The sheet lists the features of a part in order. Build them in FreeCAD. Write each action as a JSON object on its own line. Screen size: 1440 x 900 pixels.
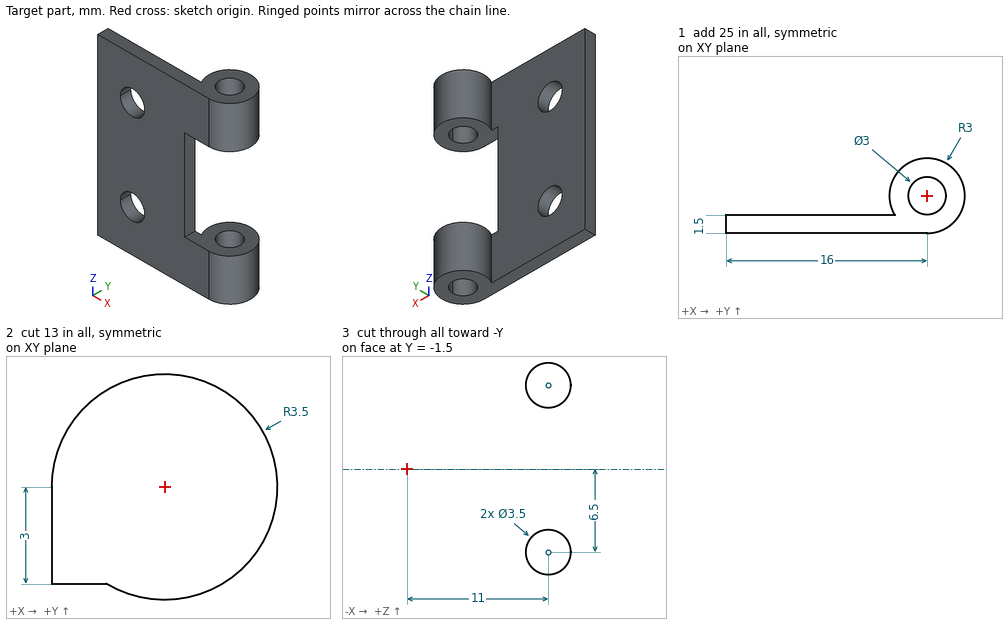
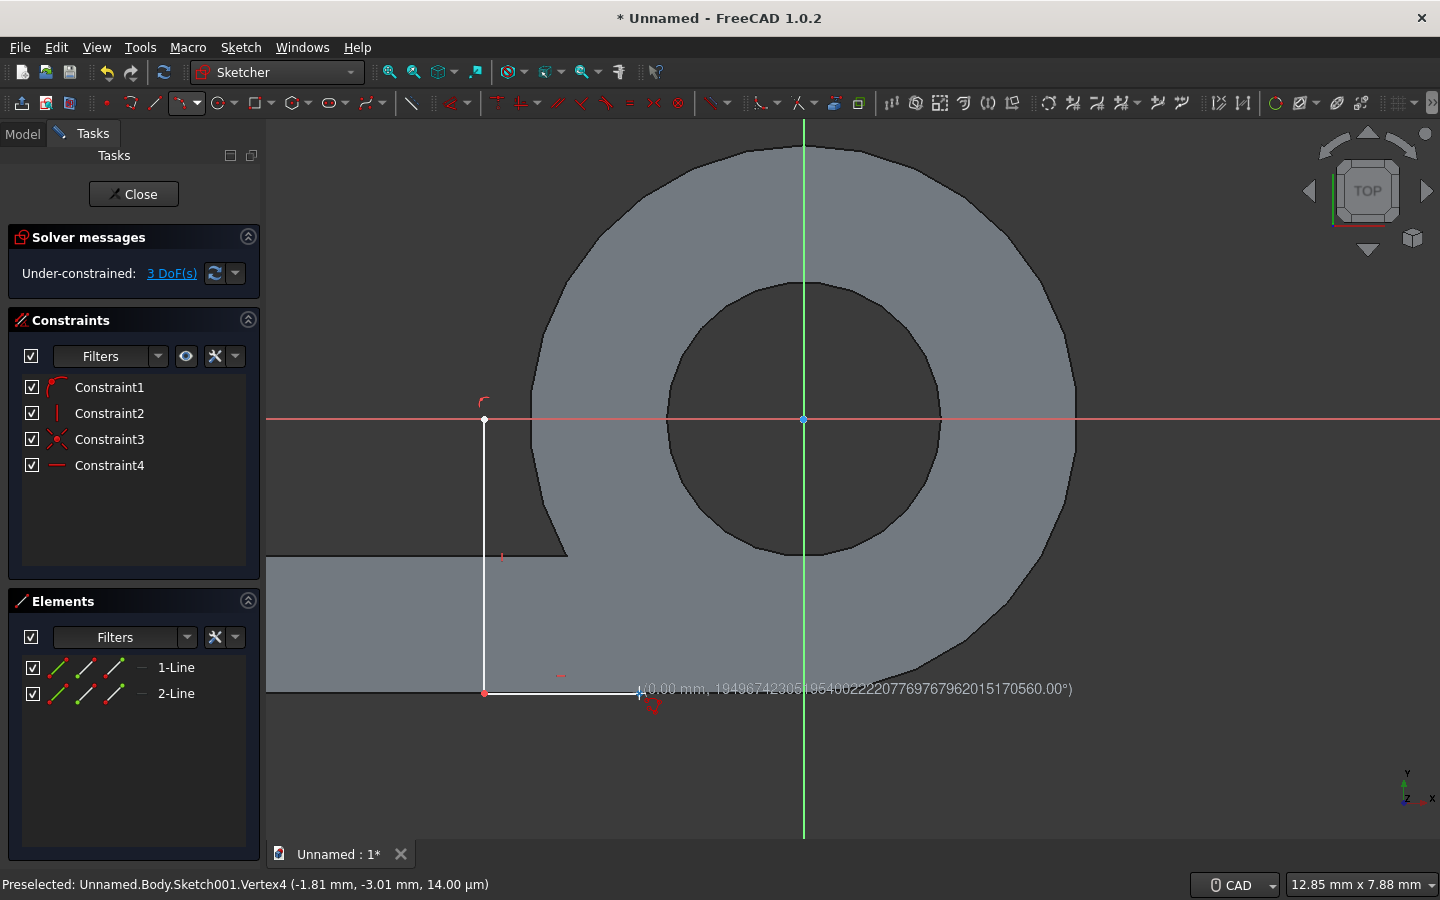
{"action": "left_click", "coordinate": [180, 104]}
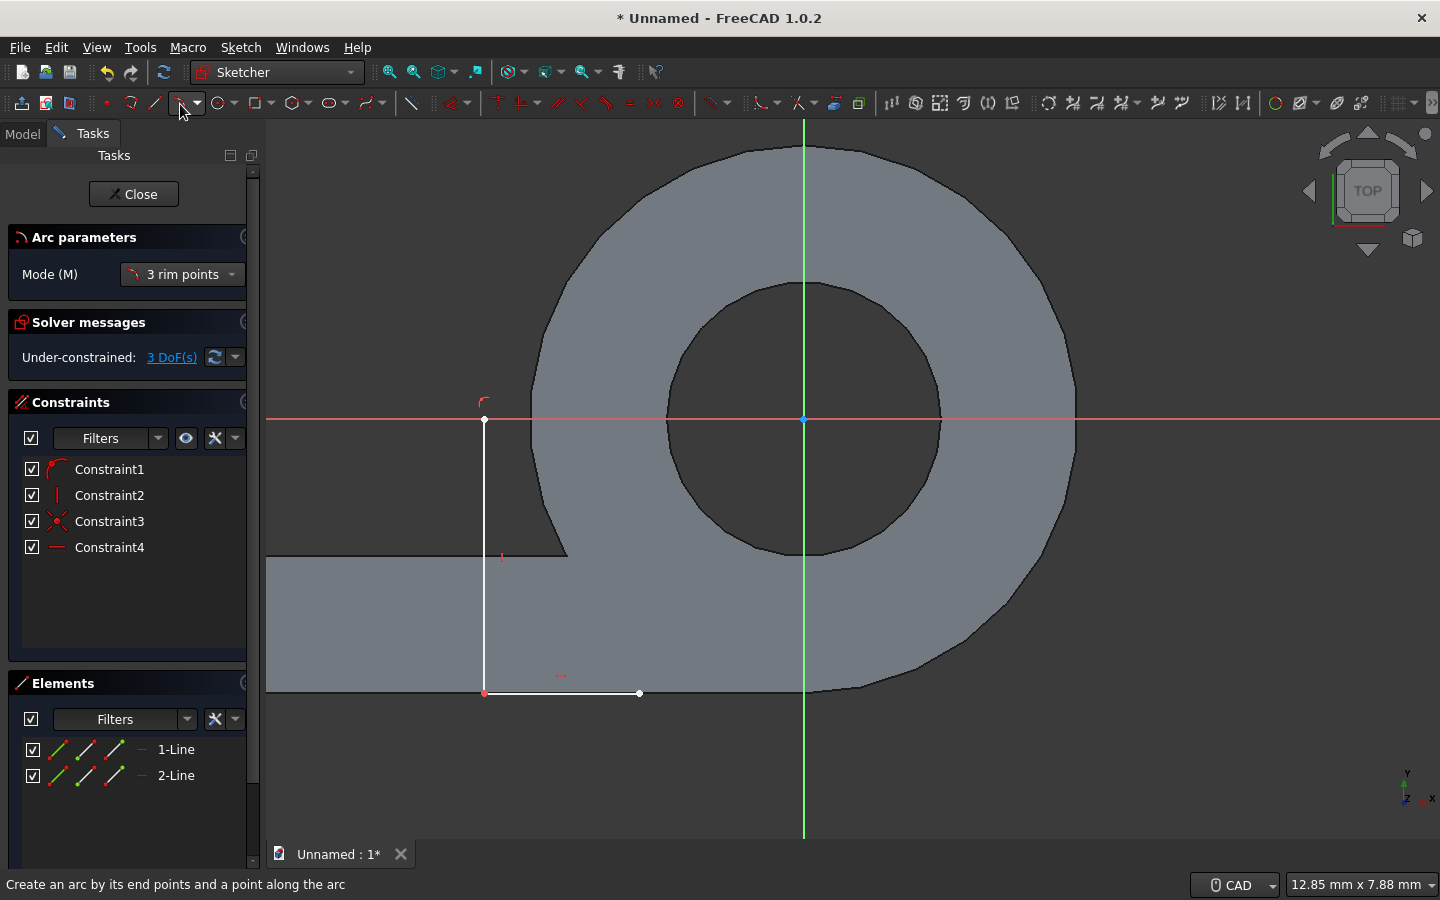
{"action": "left_click", "coordinate": [639, 694]}
{"action": "left_click", "coordinate": [484, 419]}
{"action": "left_click", "coordinate": [1082, 262]}
{"action": "key", "text": "Escape"}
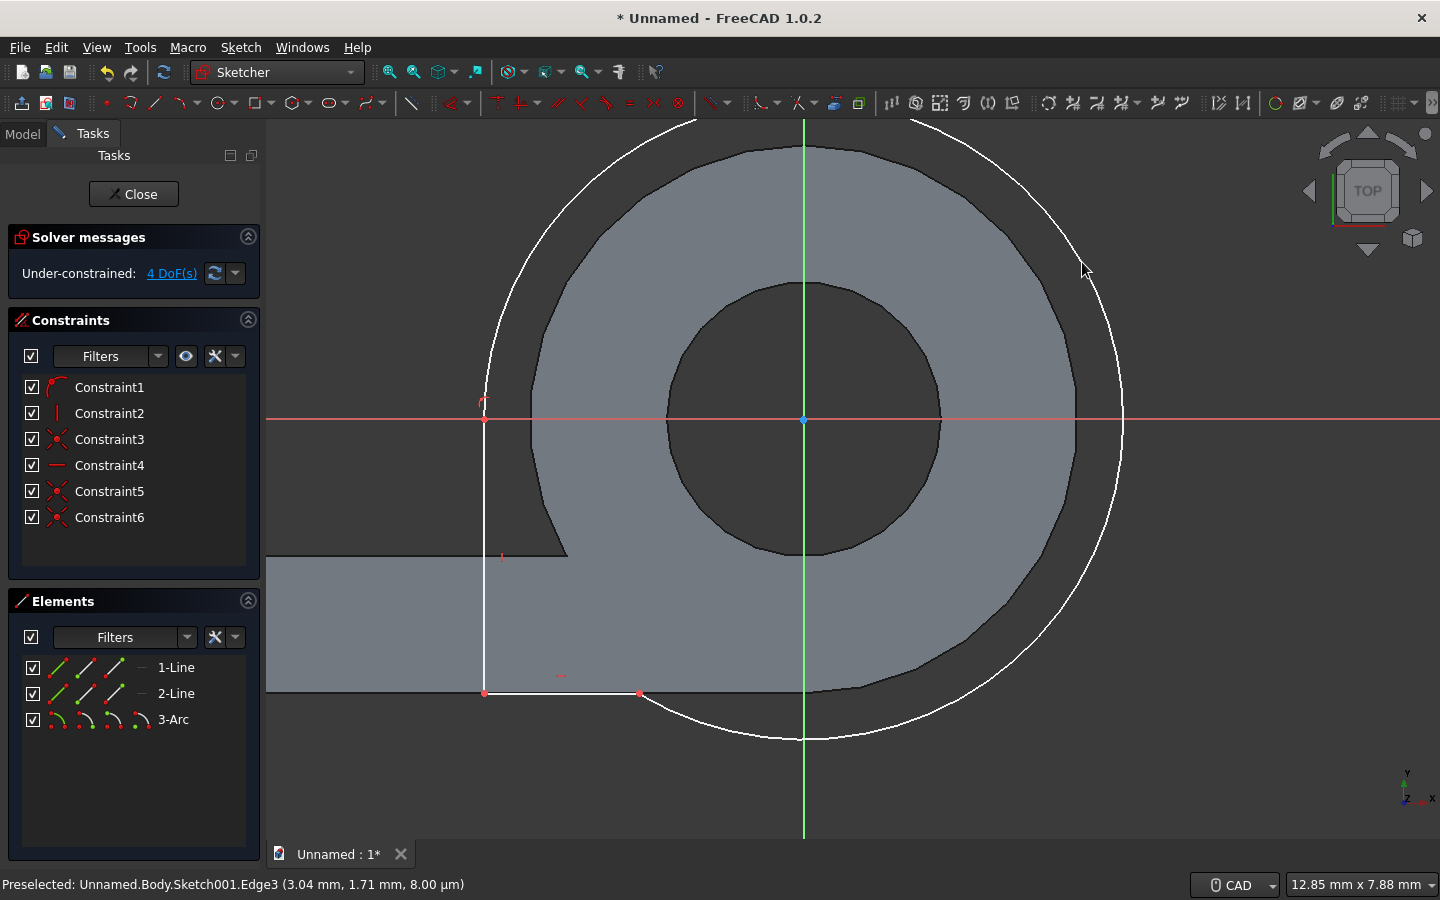
{"action": "left_click", "coordinate": [484, 502]}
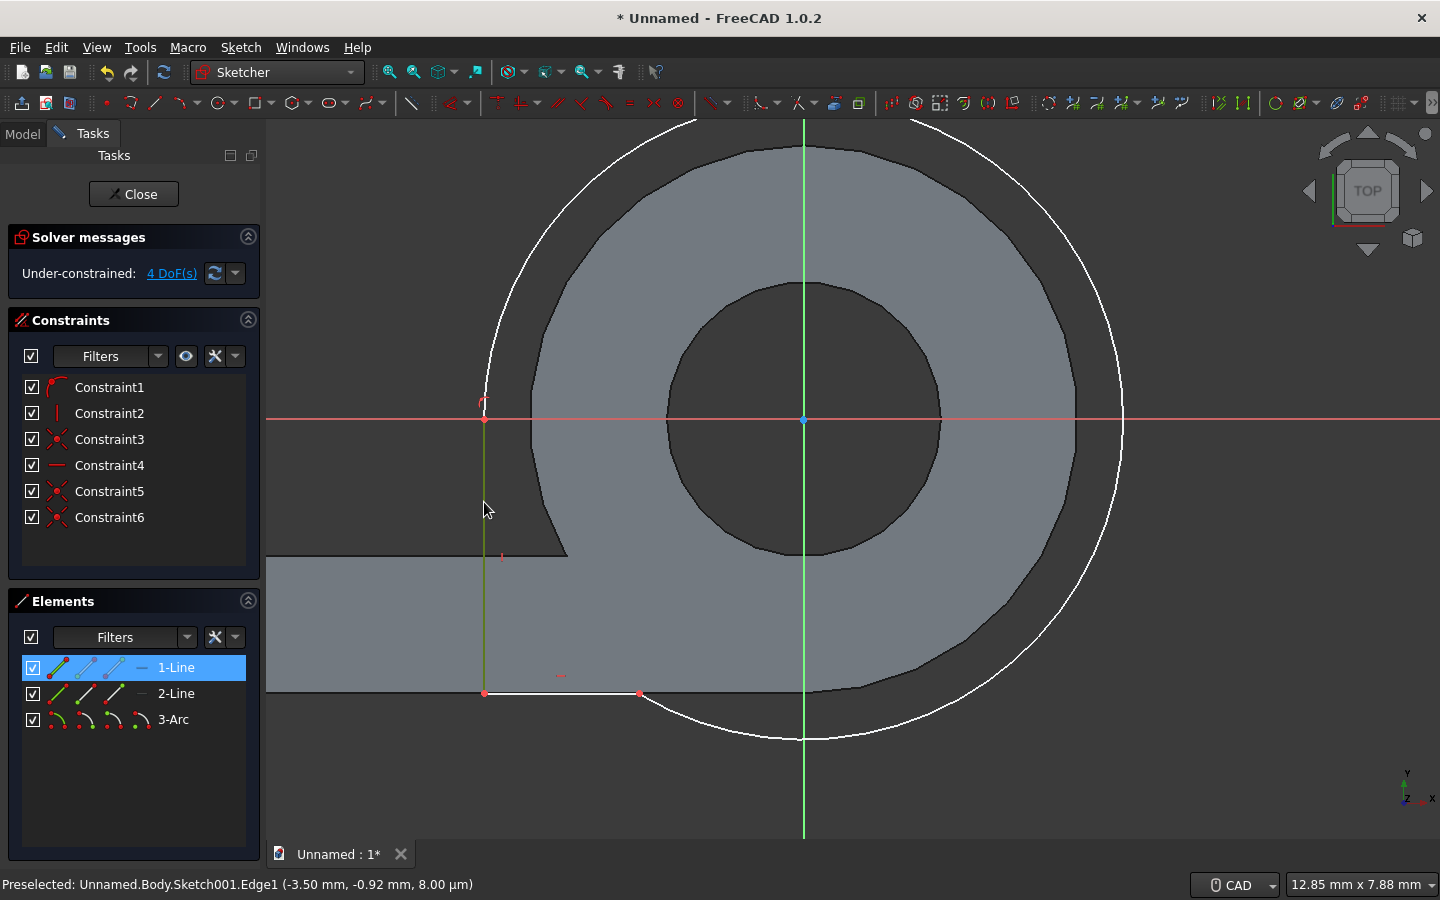
{"action": "left_click", "coordinate": [1078, 583]}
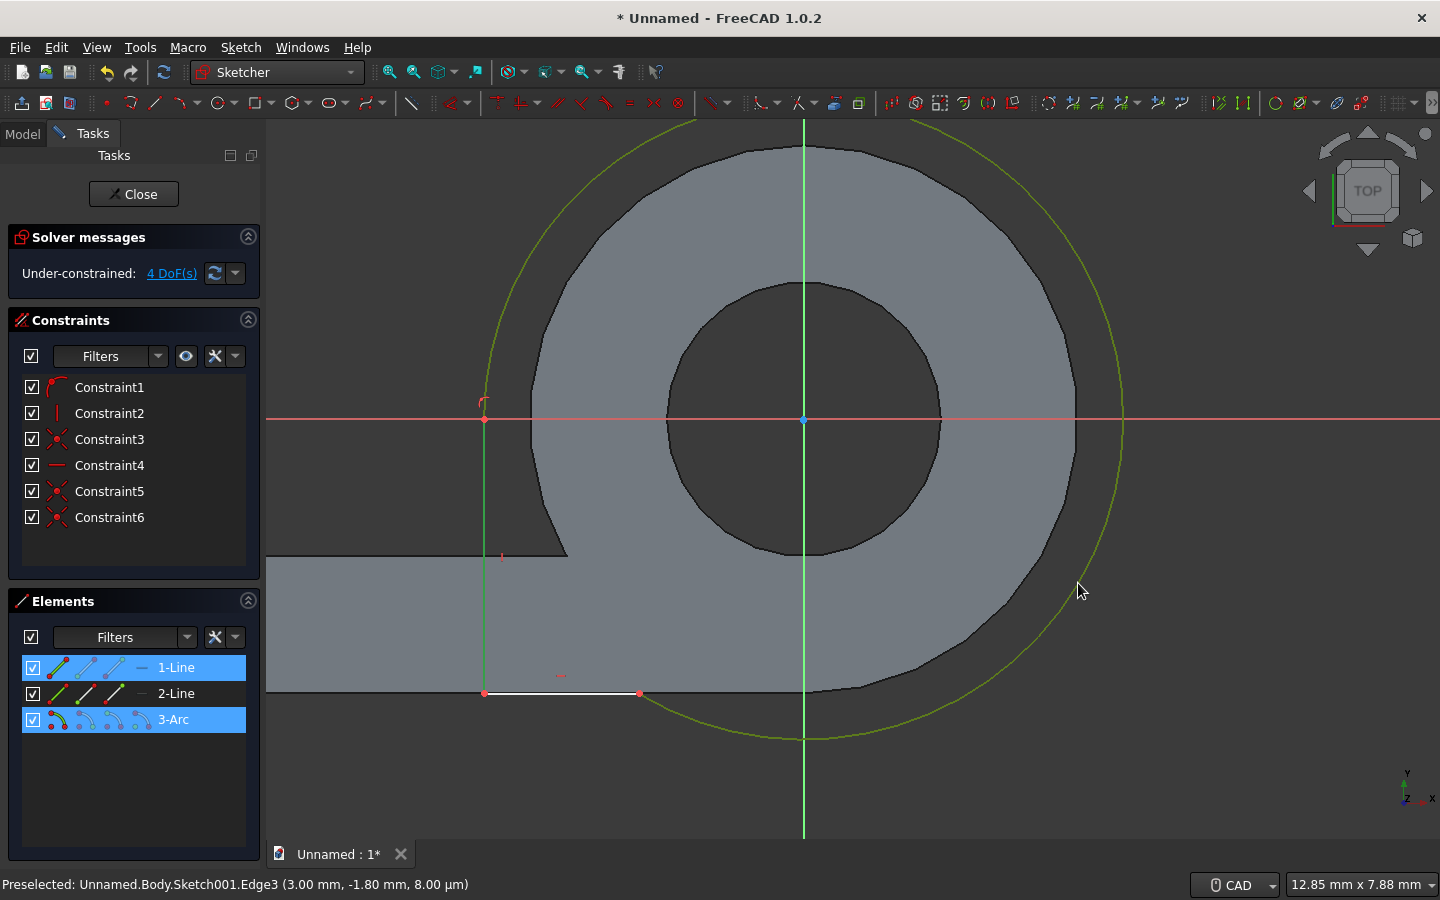
{"action": "left_click", "coordinate": [606, 104]}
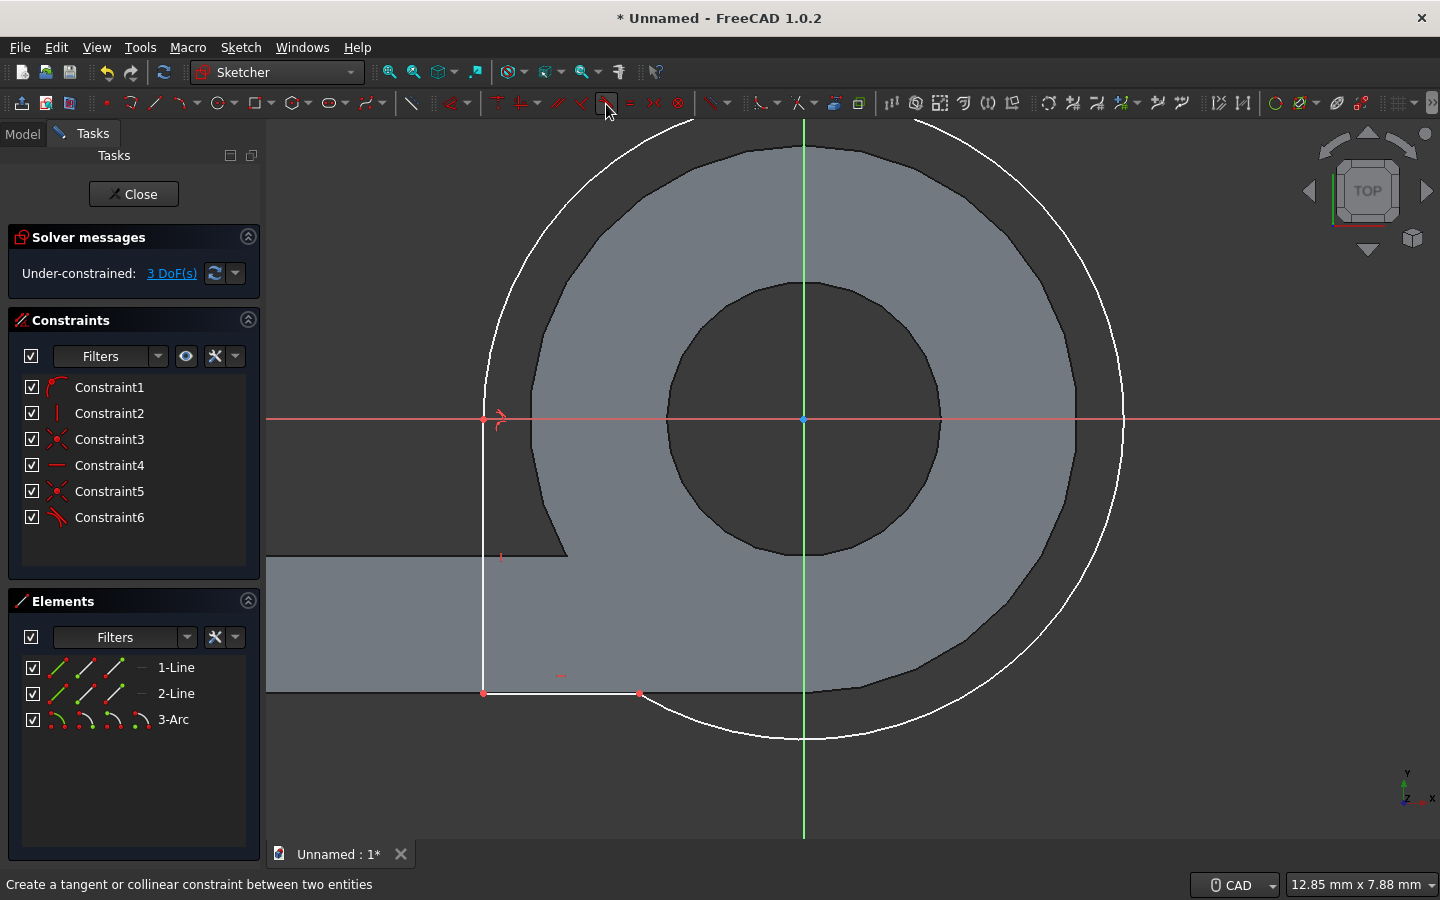
{"action": "left_click", "coordinate": [804, 419]}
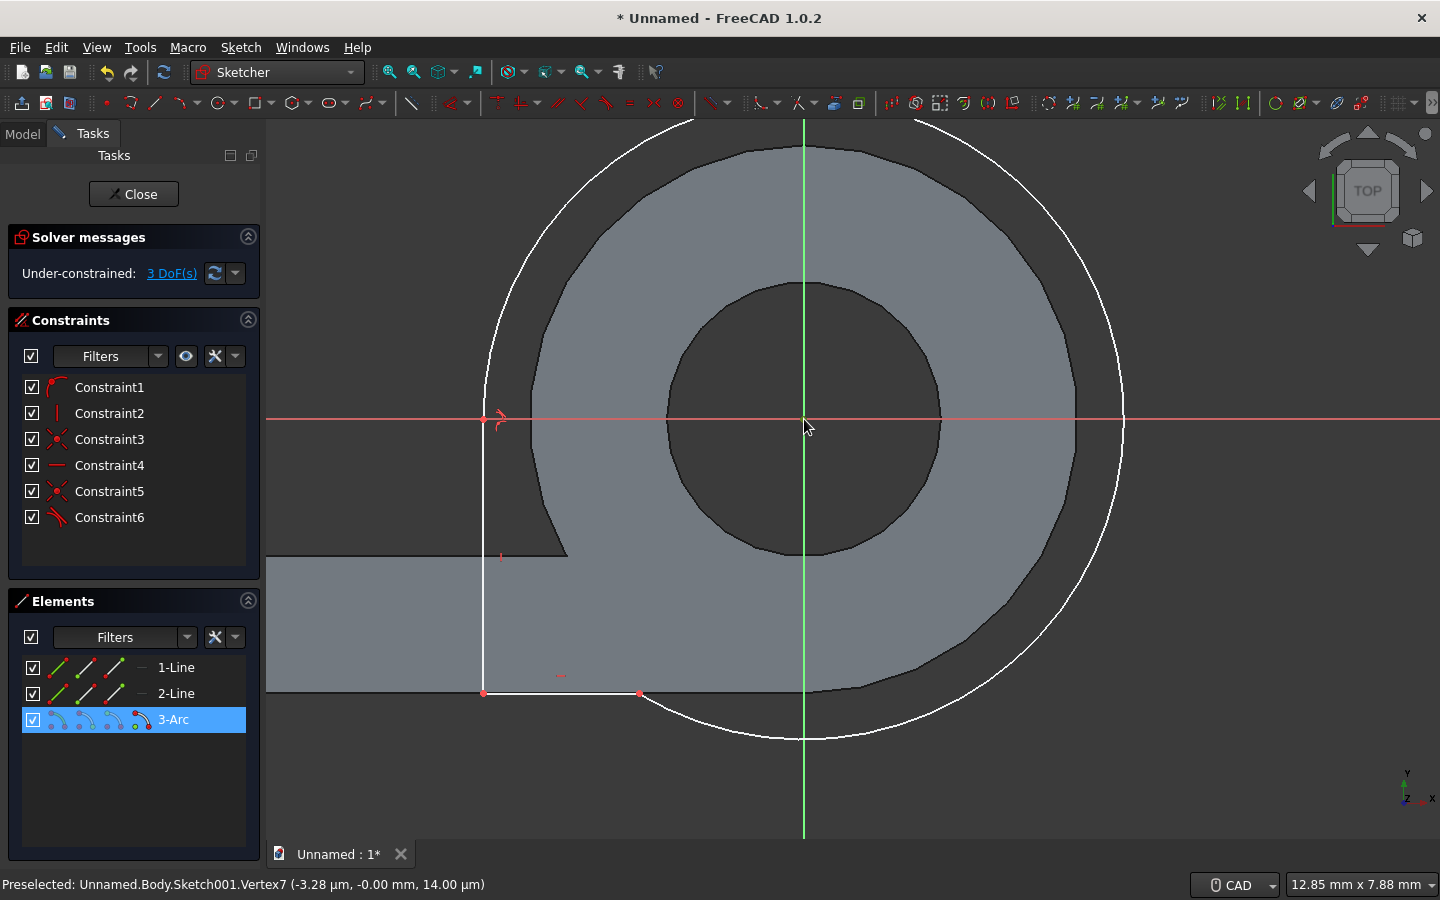
{"action": "left_click", "coordinate": [804, 669]}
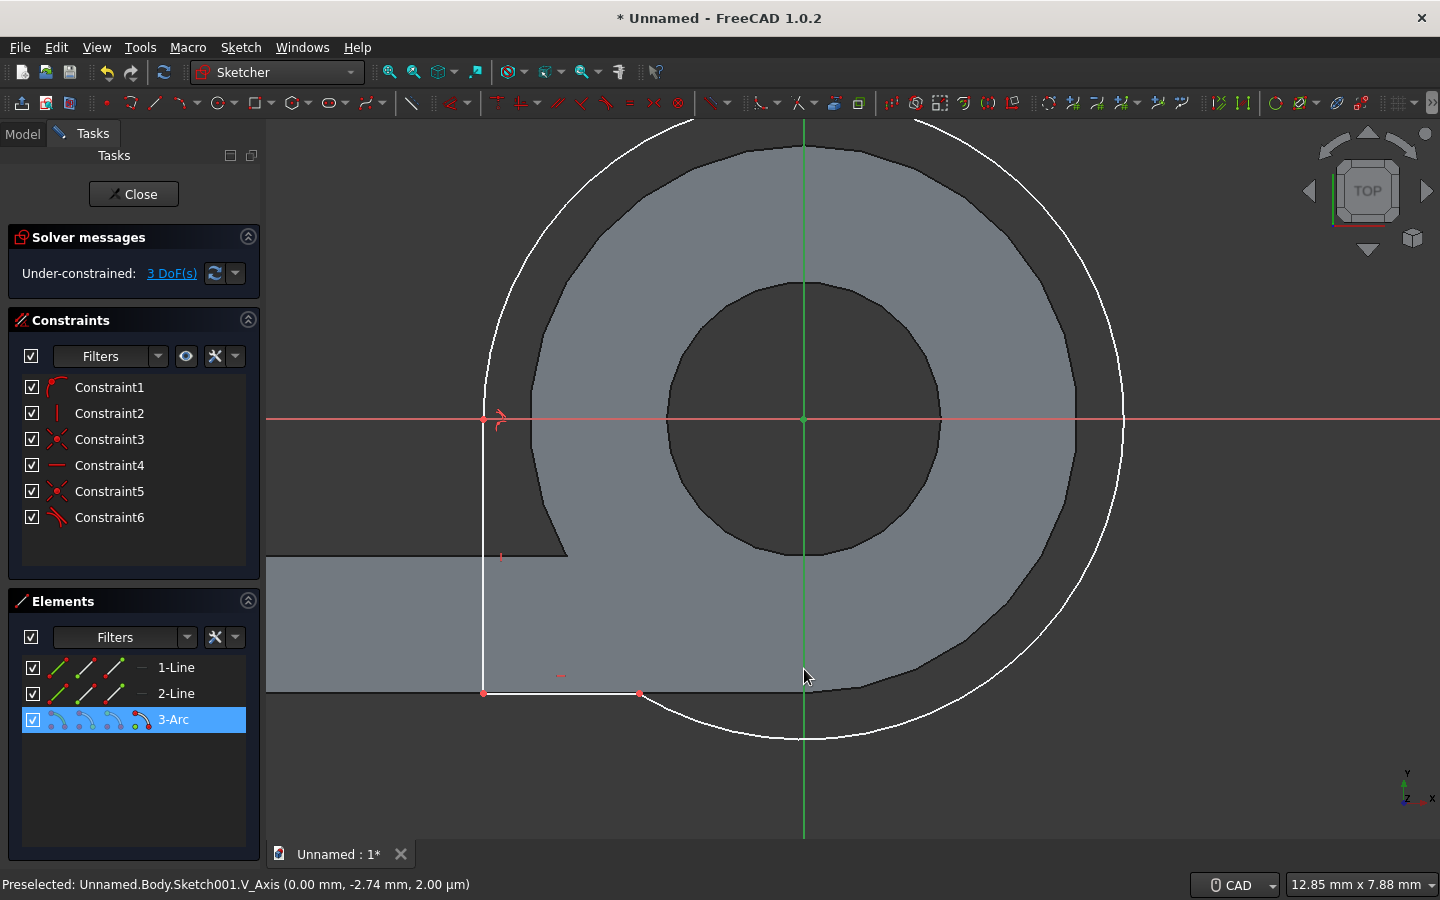
{"action": "left_click", "coordinate": [498, 104]}